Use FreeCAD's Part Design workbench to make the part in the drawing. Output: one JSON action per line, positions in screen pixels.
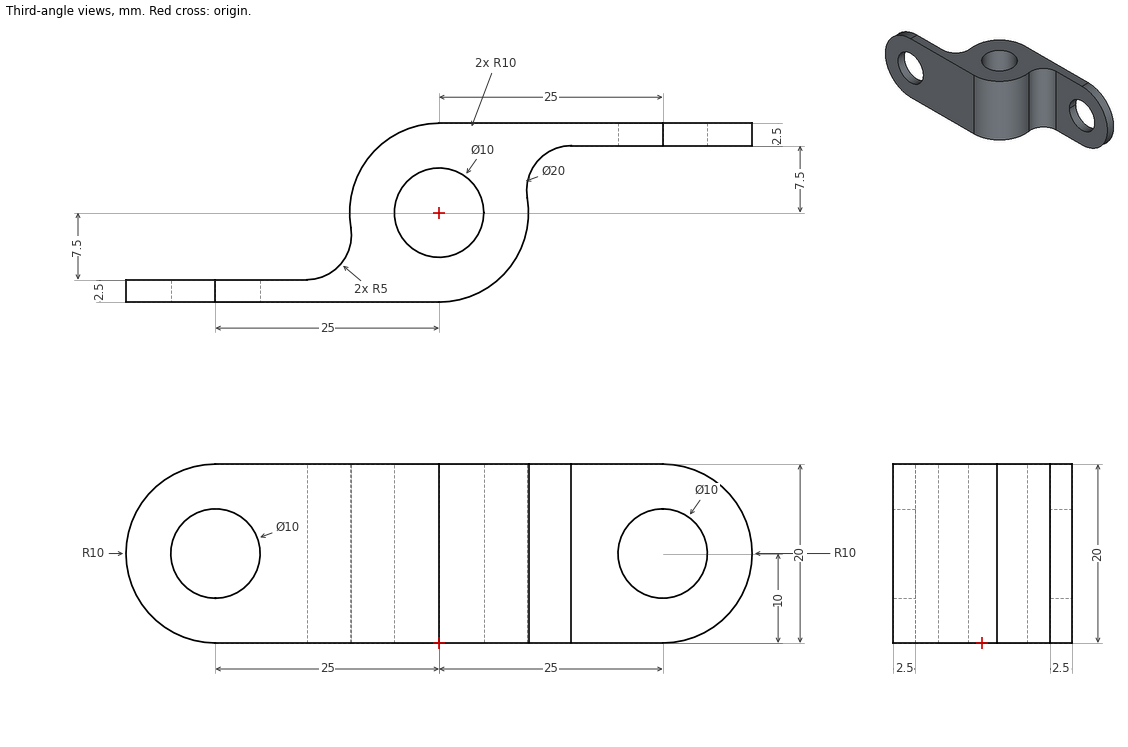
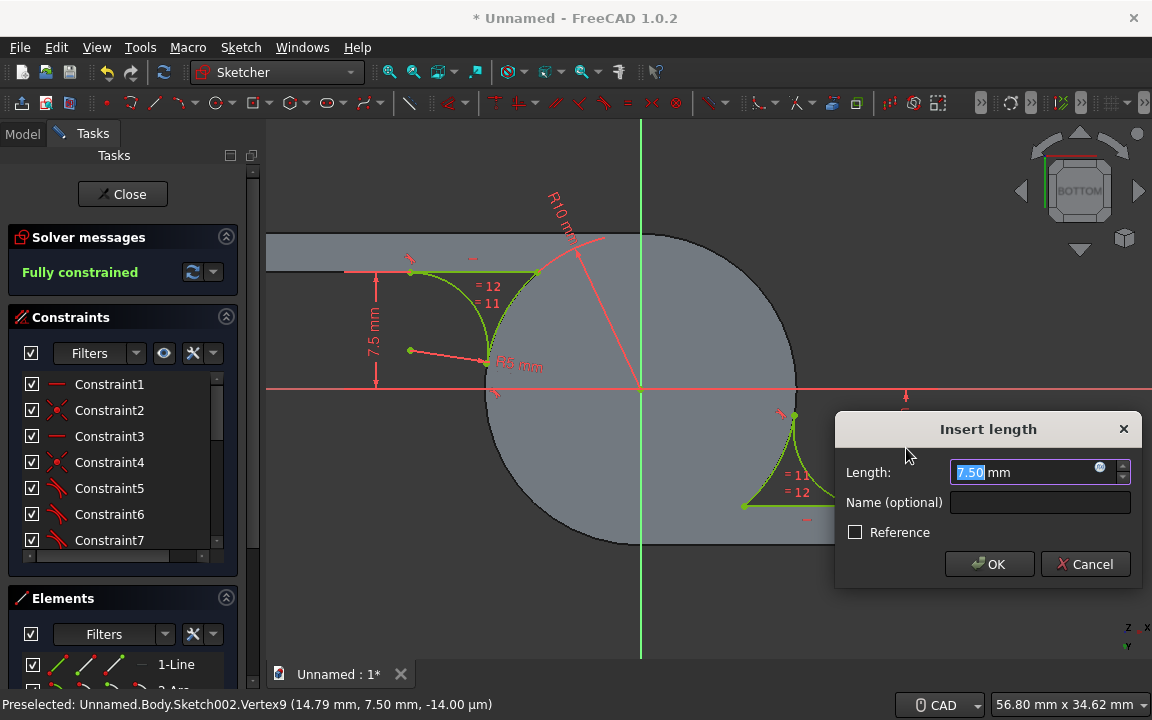
{"action": "type", "text": "7.5"}
{"action": "key", "text": "Return"}
{"action": "key", "text": "Escape"}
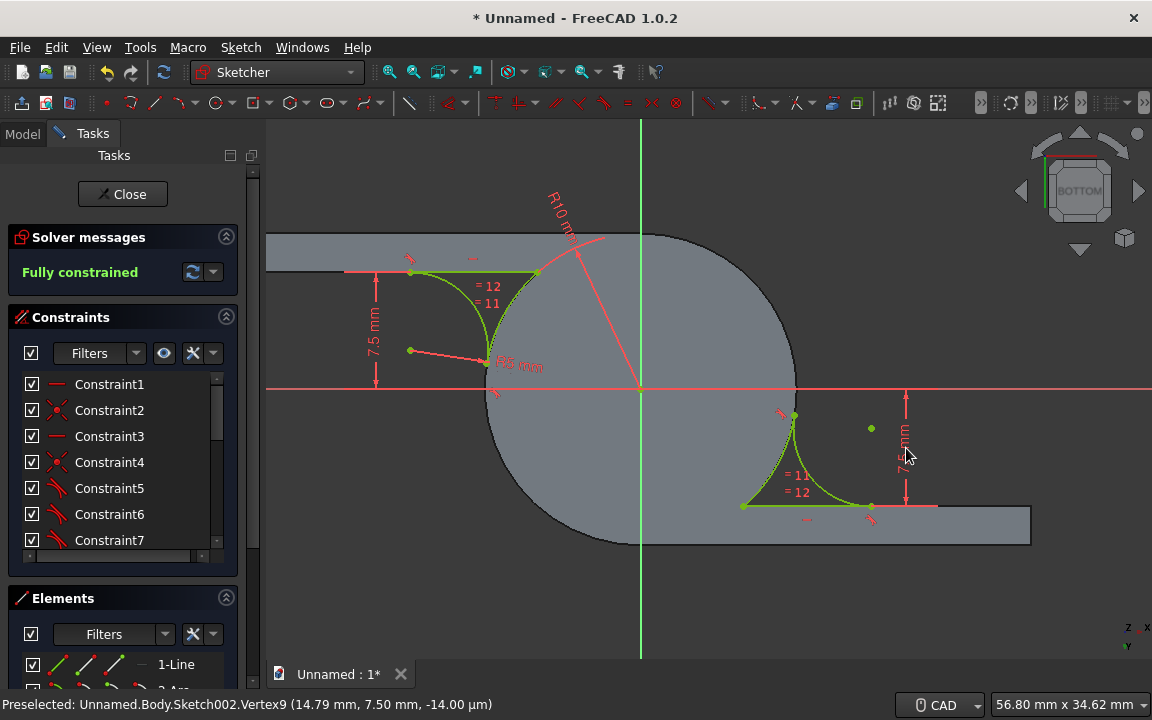
{"action": "left_click", "coordinate": [123, 194]}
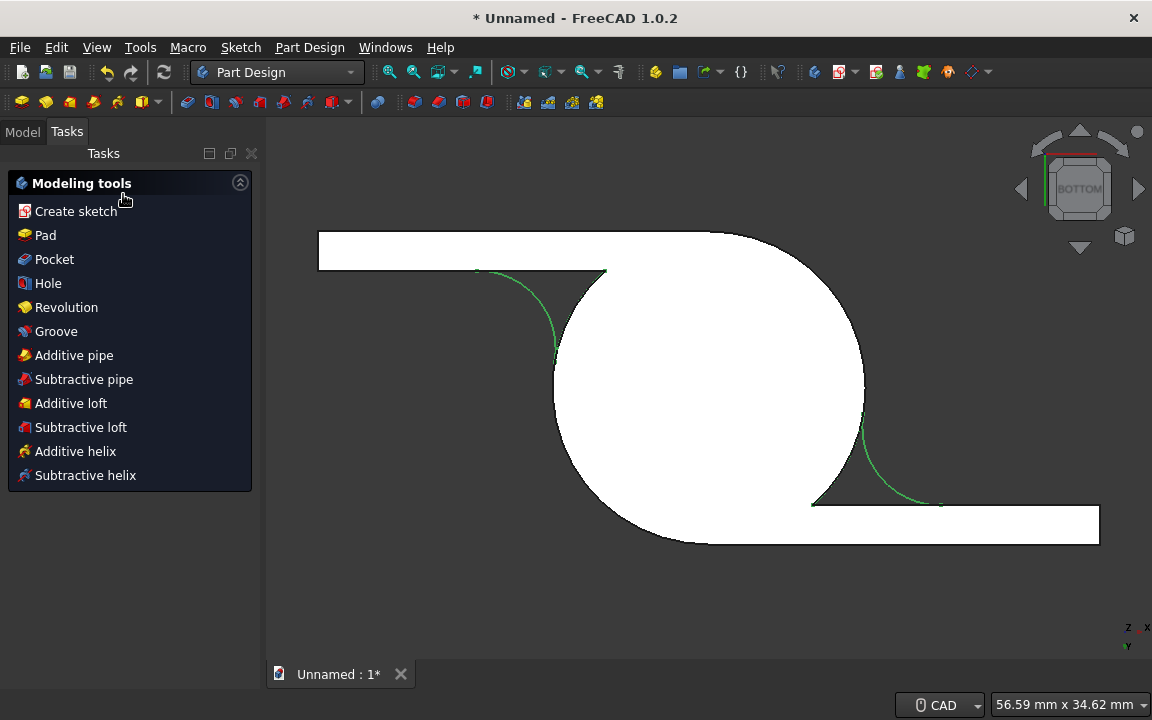
{"action": "left_click", "coordinate": [22, 102]}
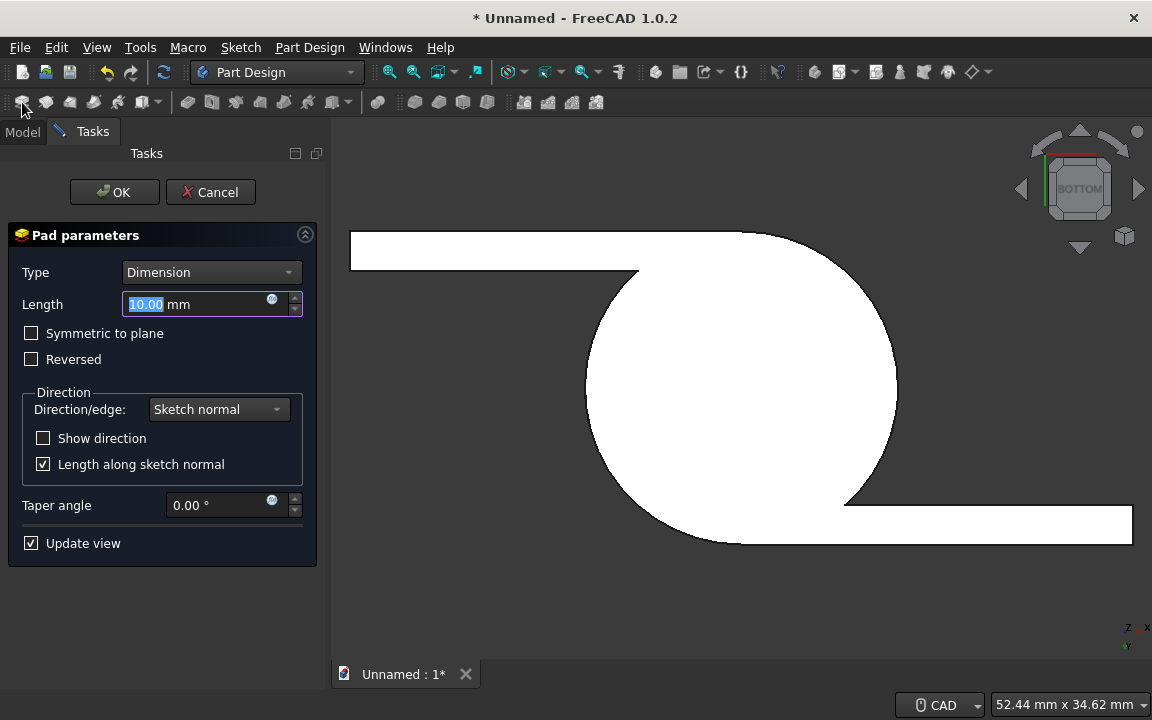
{"action": "type", "text": "20"}
{"action": "key", "text": "Tab"}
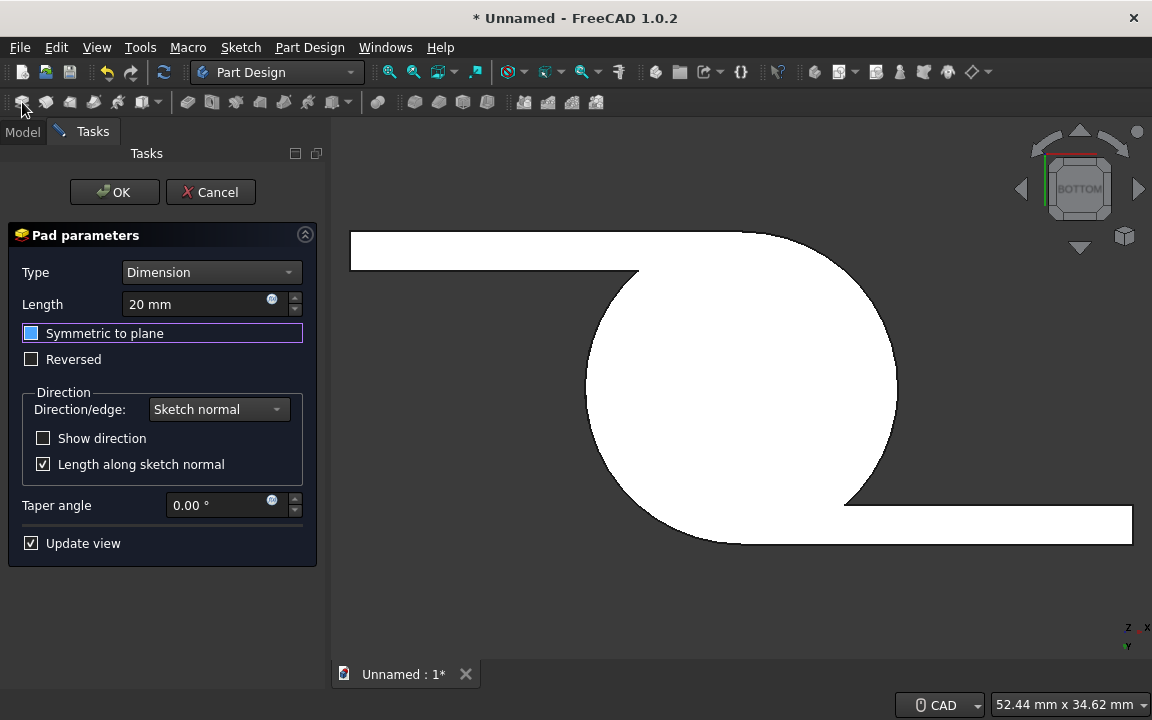
{"action": "left_click", "coordinate": [30, 359]}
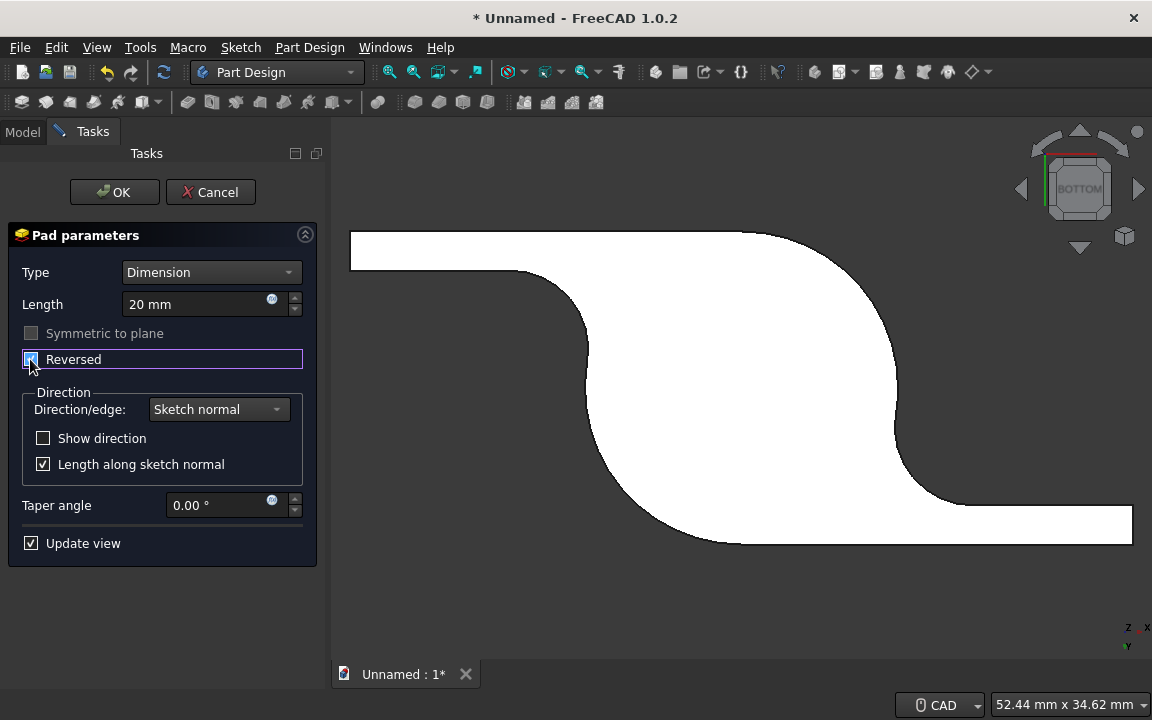
{"action": "left_click", "coordinate": [115, 192]}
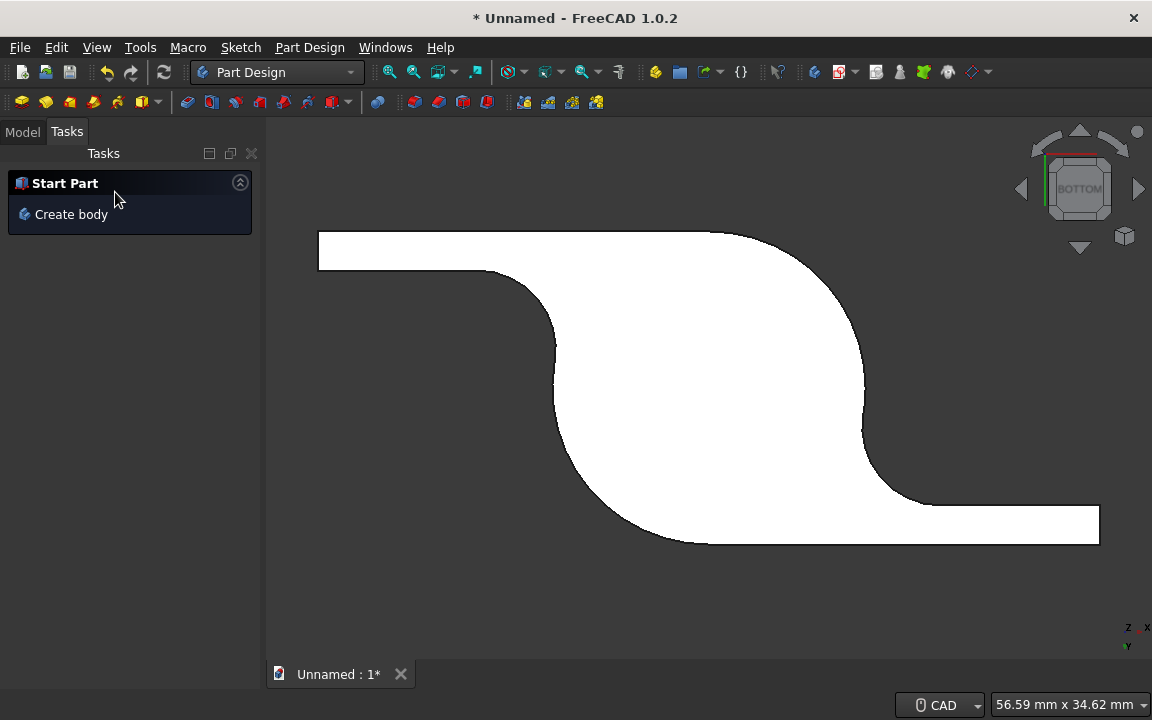
{"action": "key", "text": "0"}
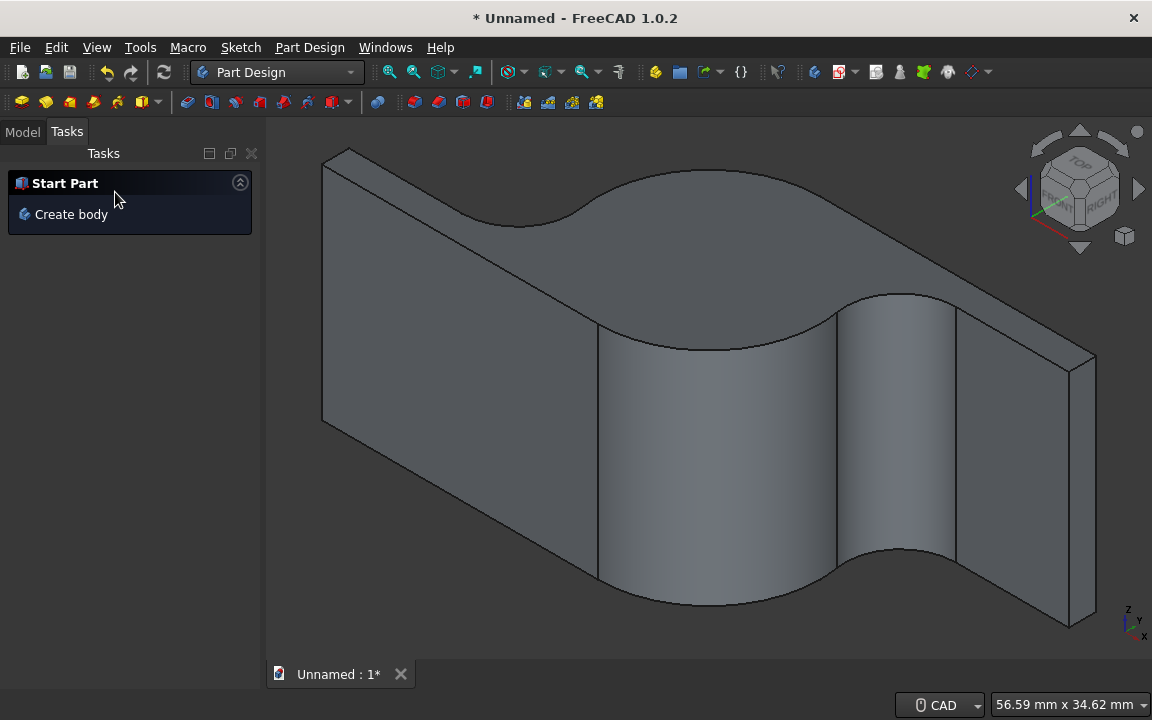
{"action": "left_click", "coordinate": [390, 72]}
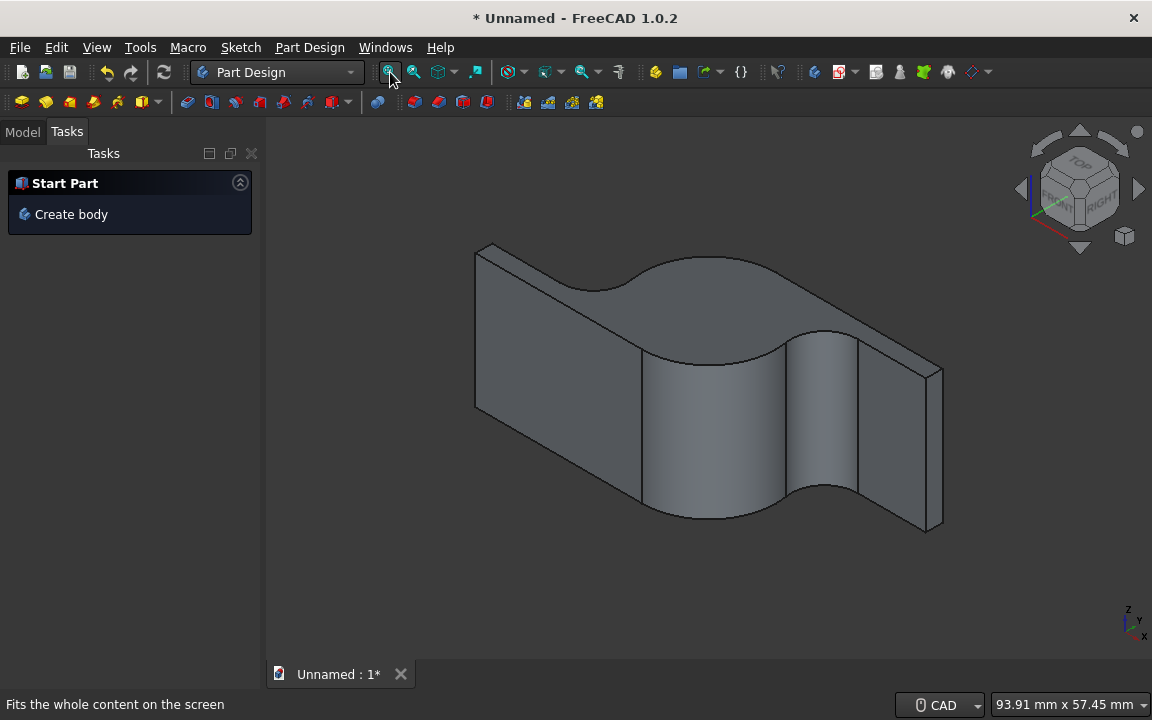
{"action": "left_click", "coordinate": [559, 377]}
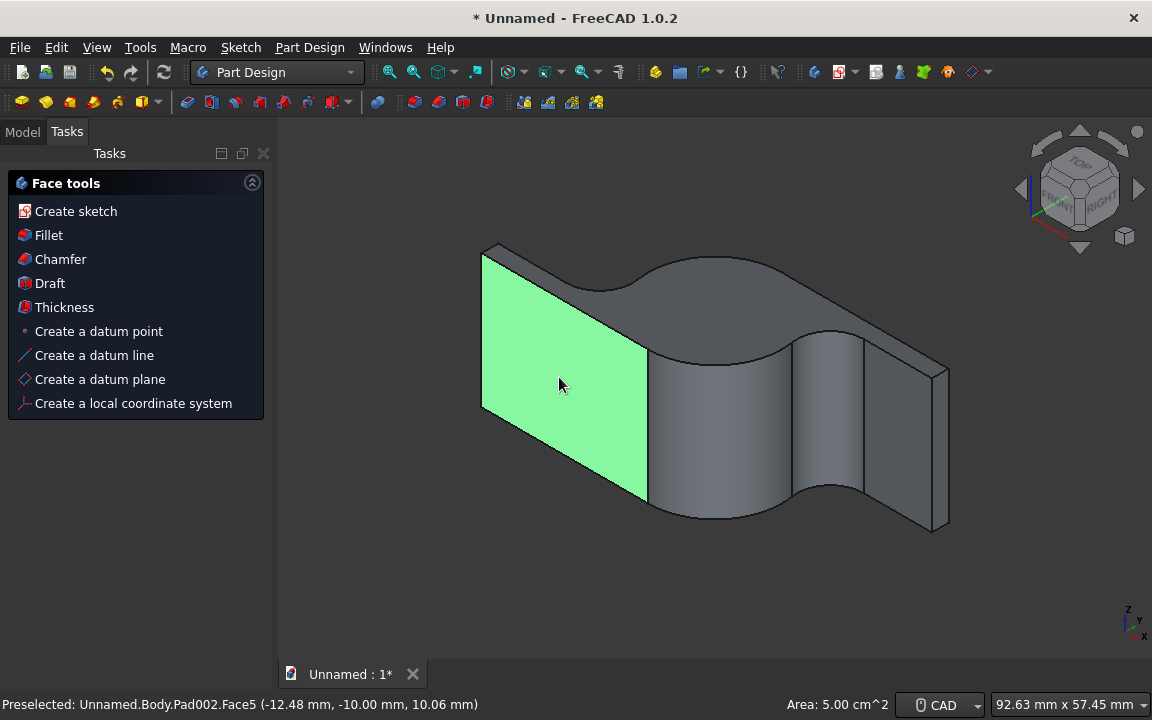
{"action": "left_click", "coordinate": [840, 72]}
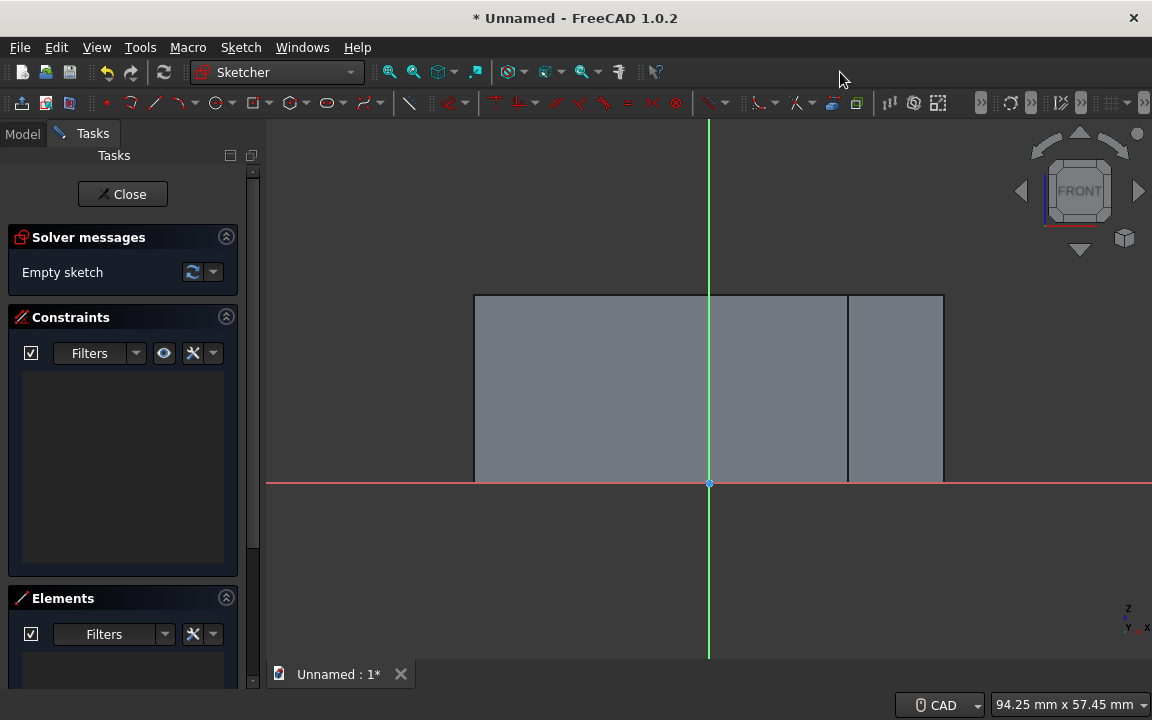
{"action": "scroll", "coordinate": [349, 389], "scroll_direction": "up", "scroll_amount": 2}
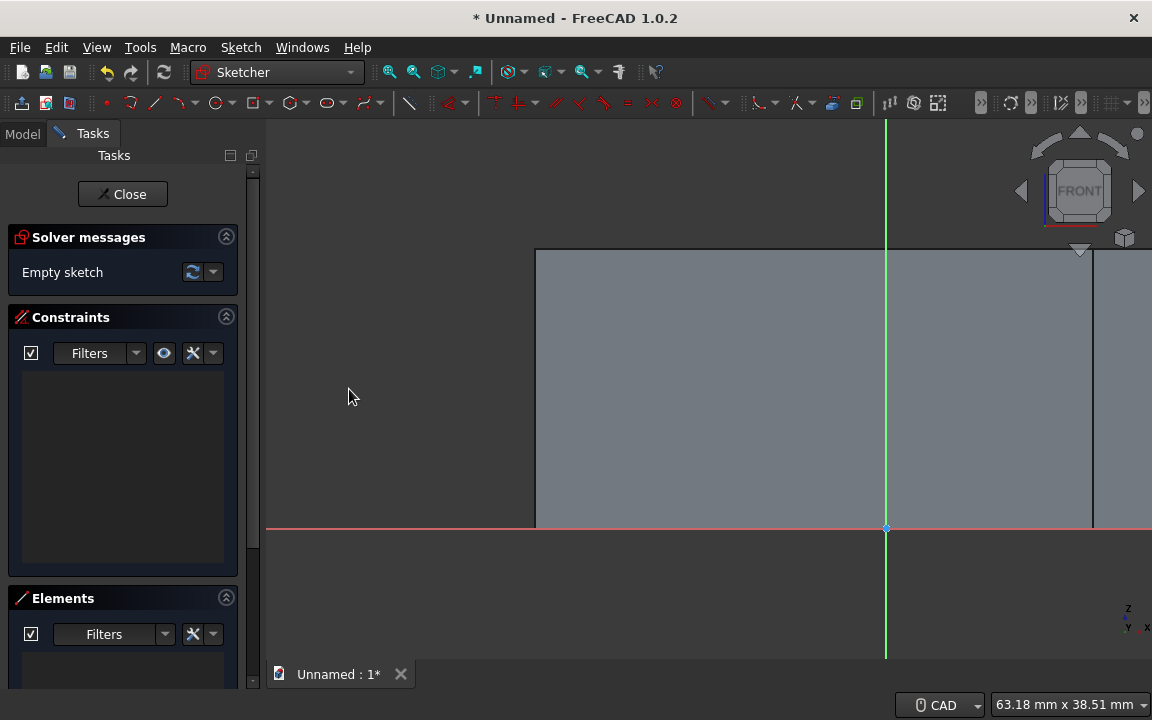
{"action": "key", "text": "g l"}